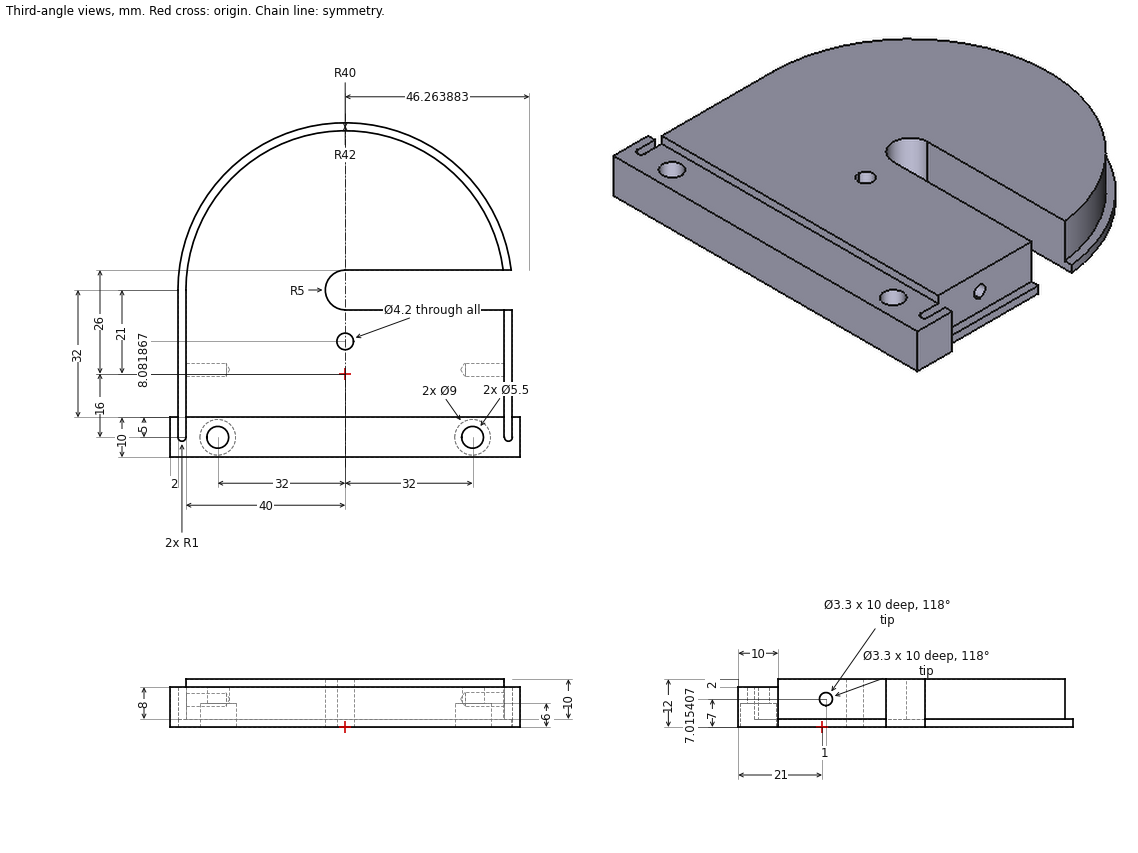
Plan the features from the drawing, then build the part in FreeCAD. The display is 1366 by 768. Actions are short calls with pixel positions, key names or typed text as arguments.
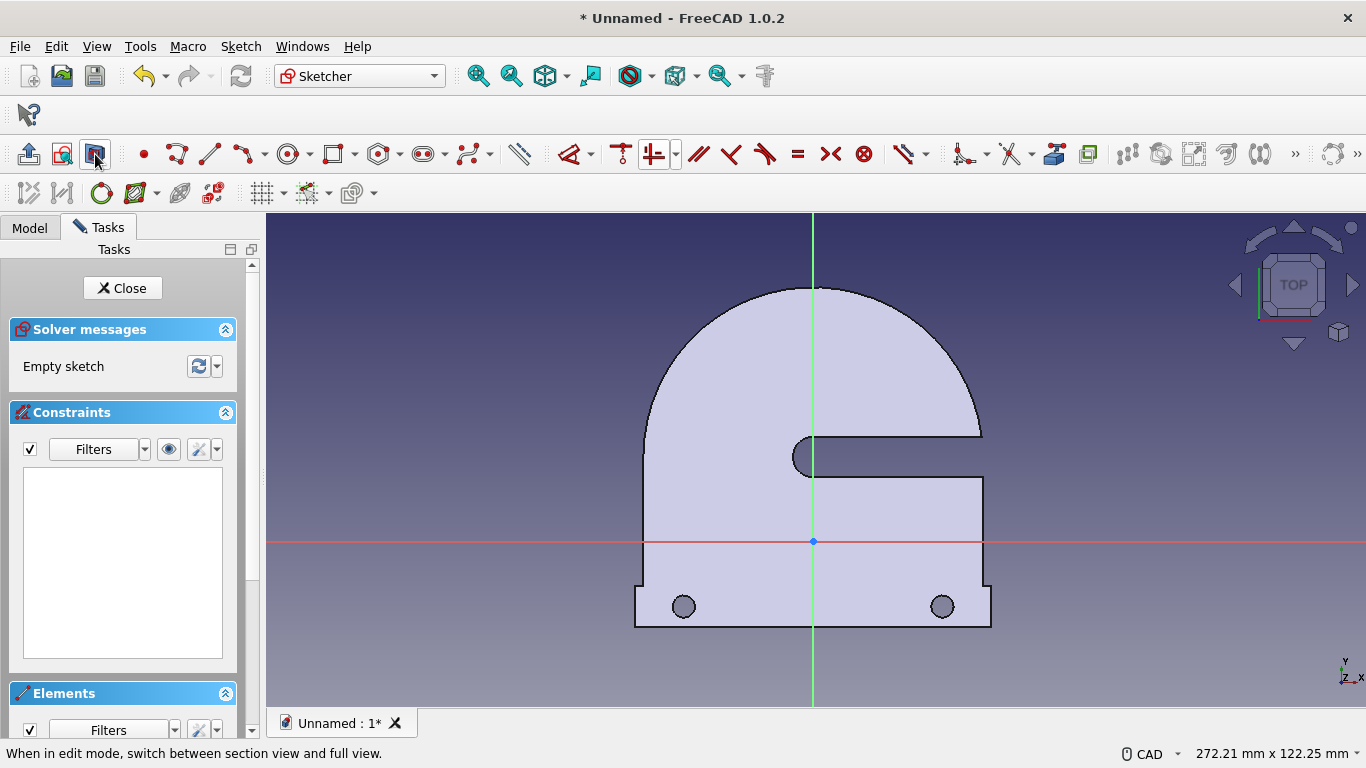
scroll(867, 679, up, 4)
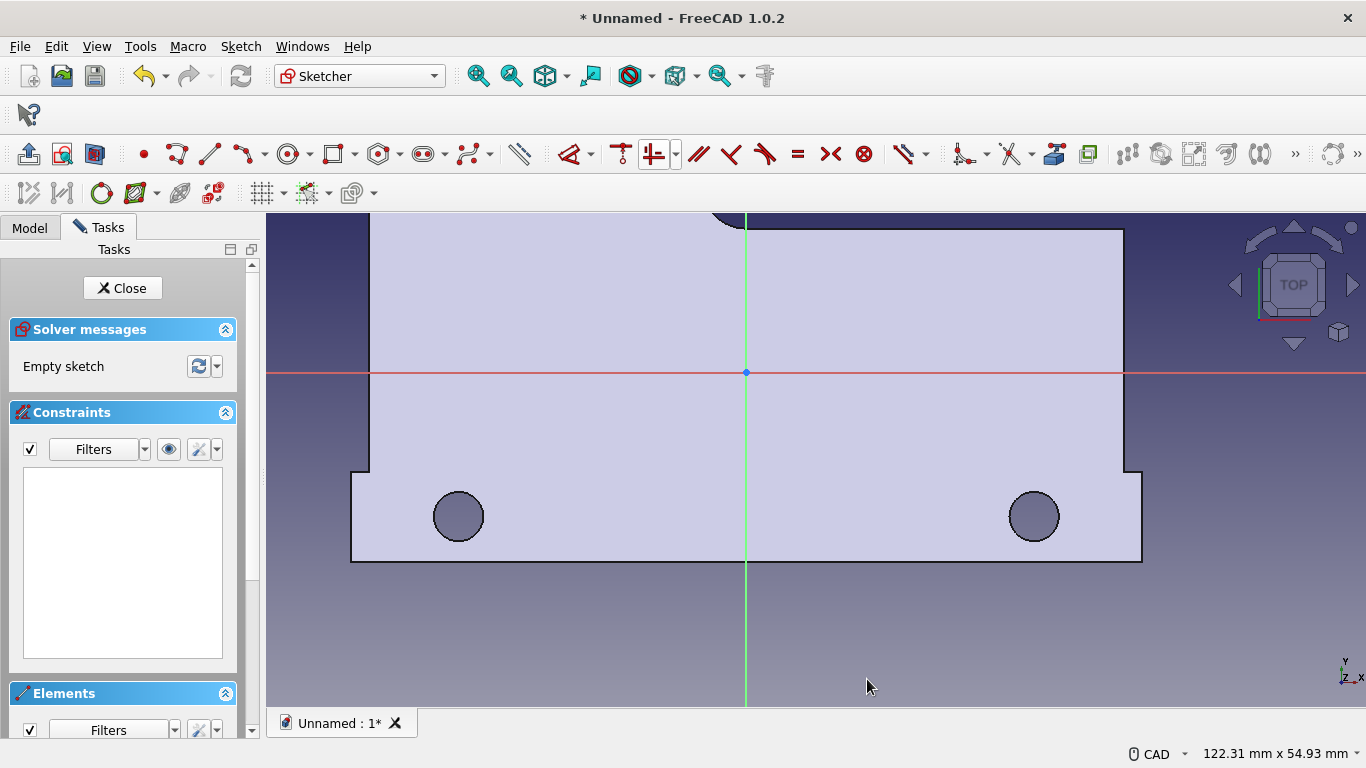
click(288, 154)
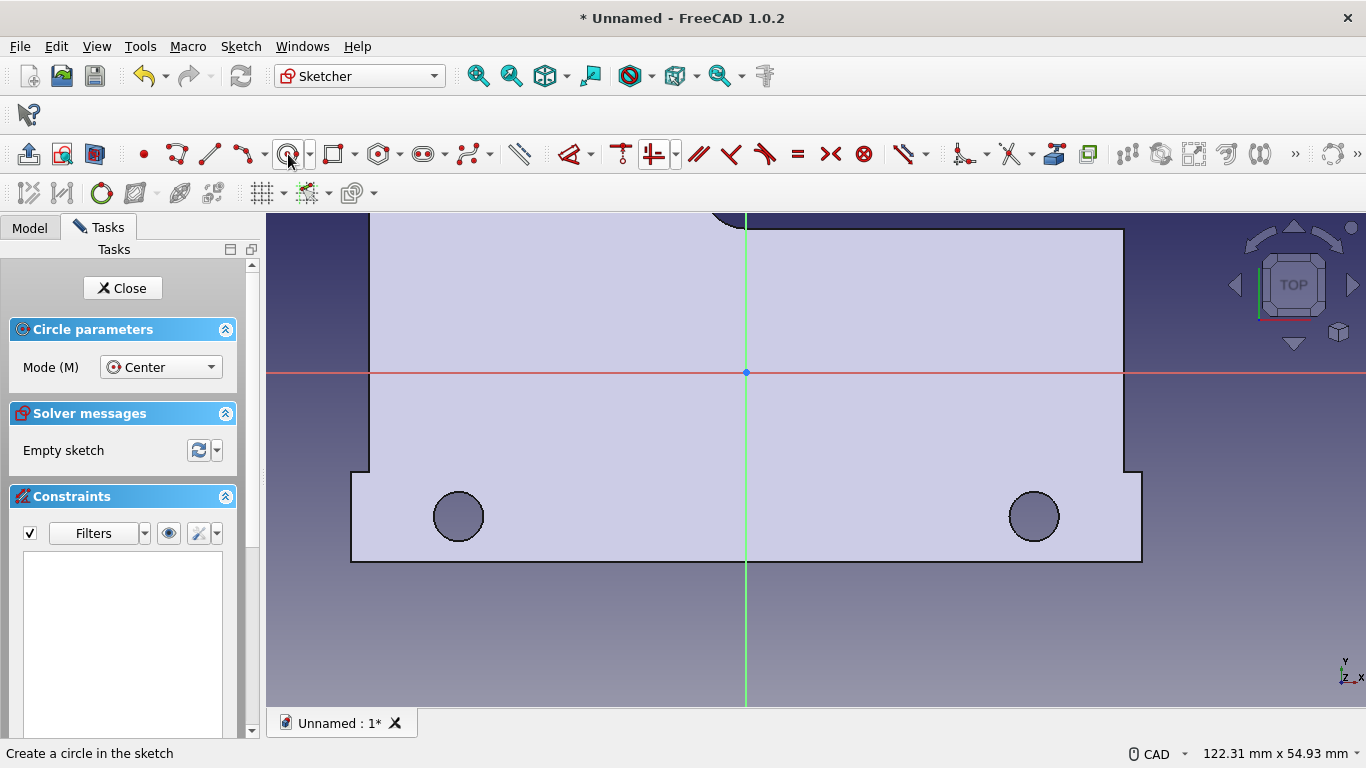
click(1034, 517)
click(1063, 488)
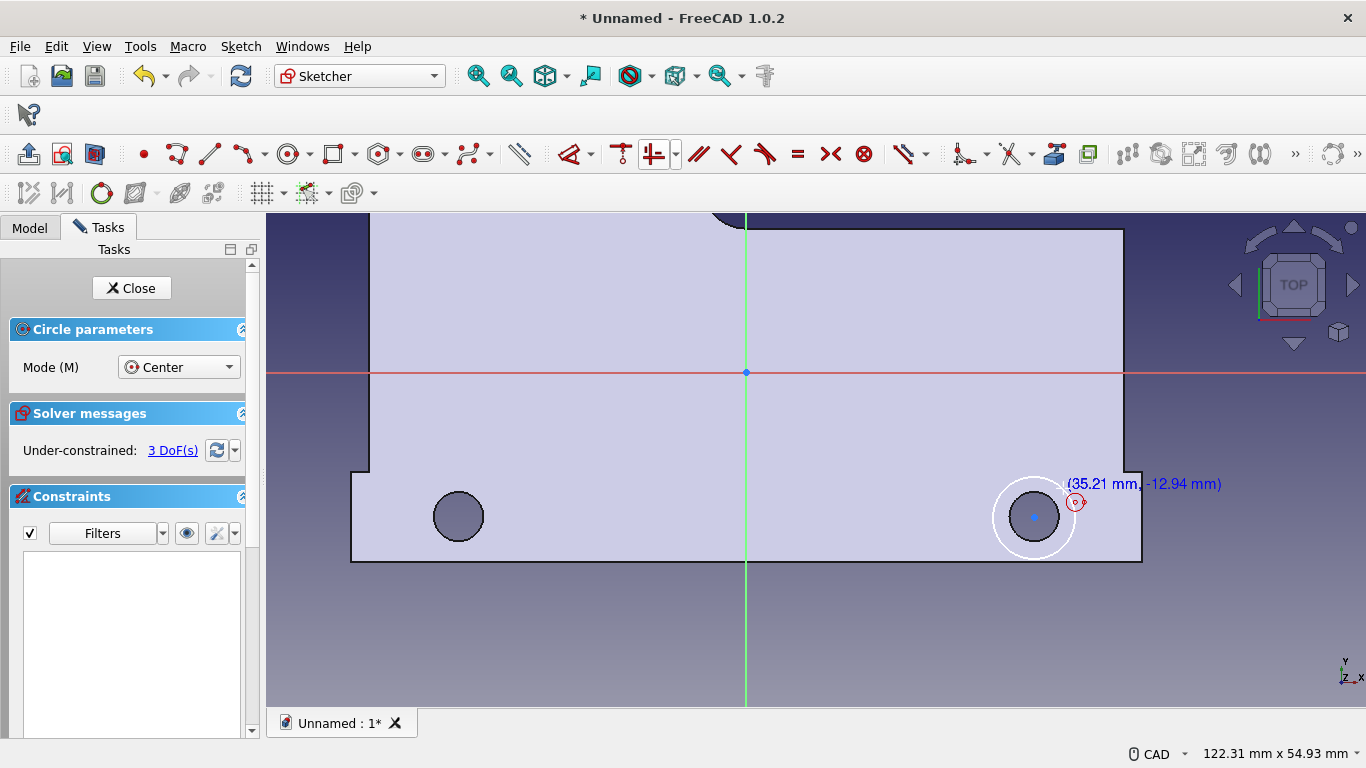
click(459, 517)
click(487, 488)
key(Escape)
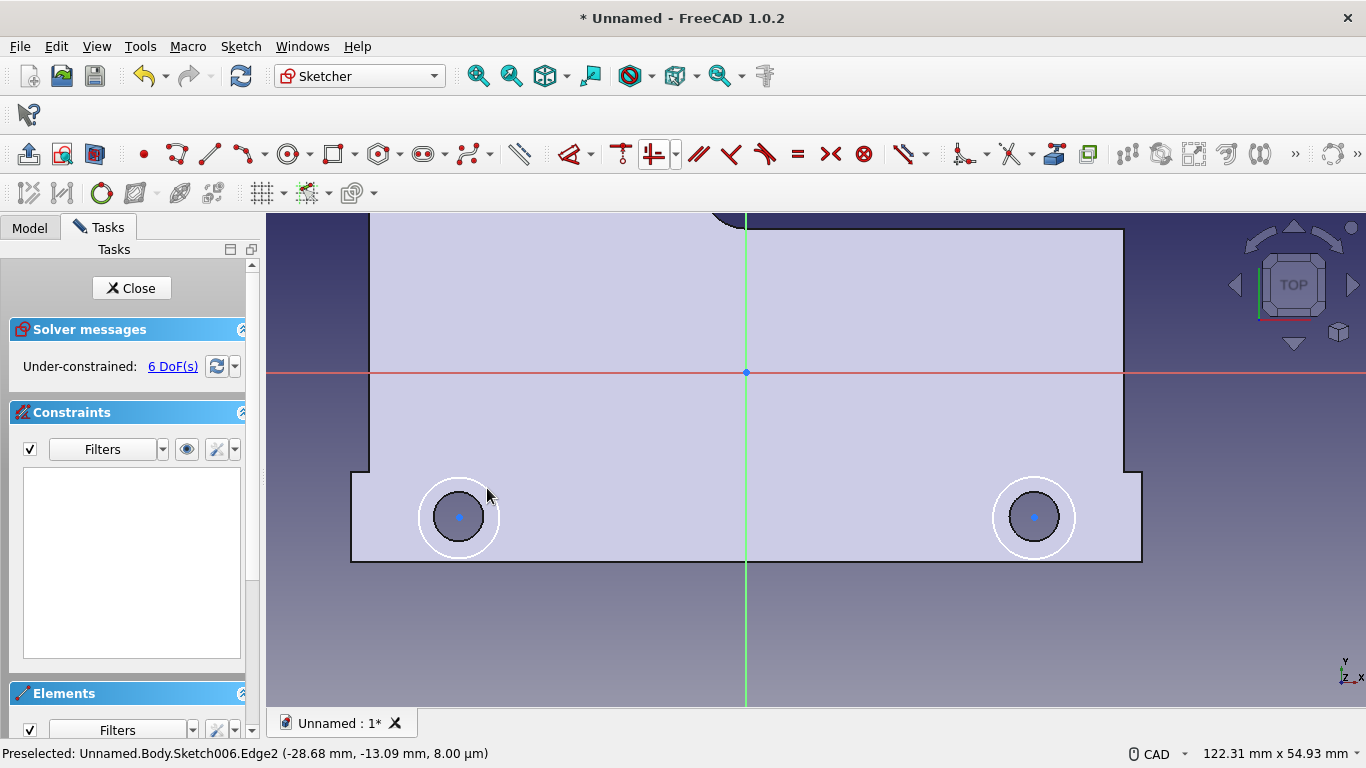
click(1063, 489)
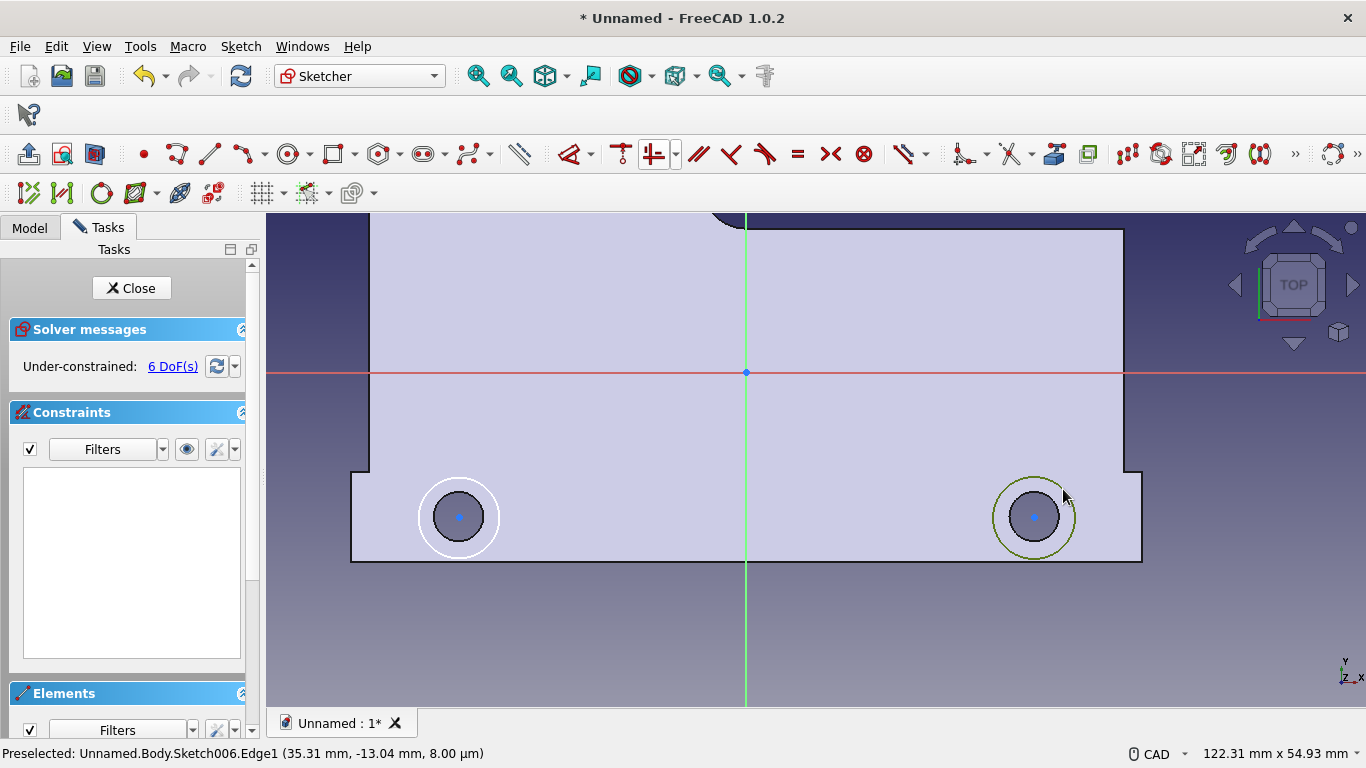
click(487, 489)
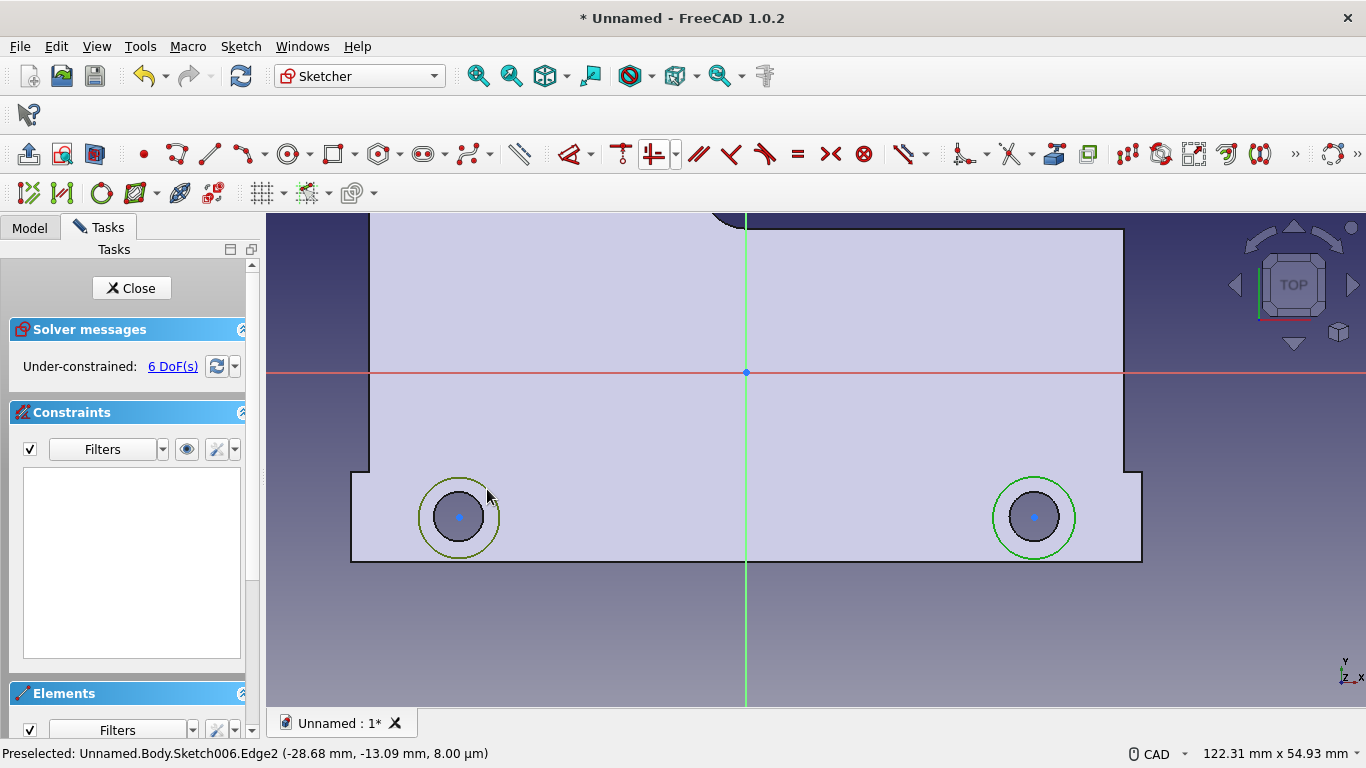
click(798, 154)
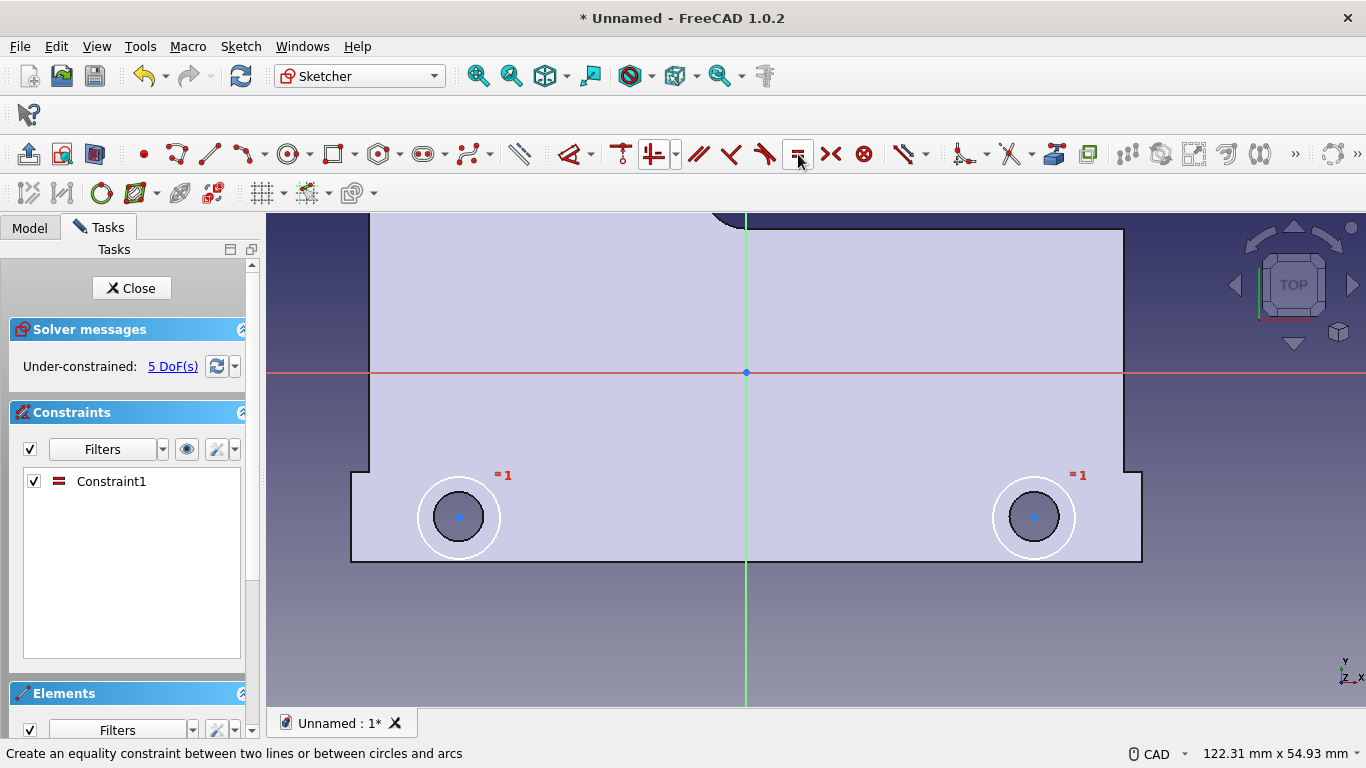
click(1034, 518)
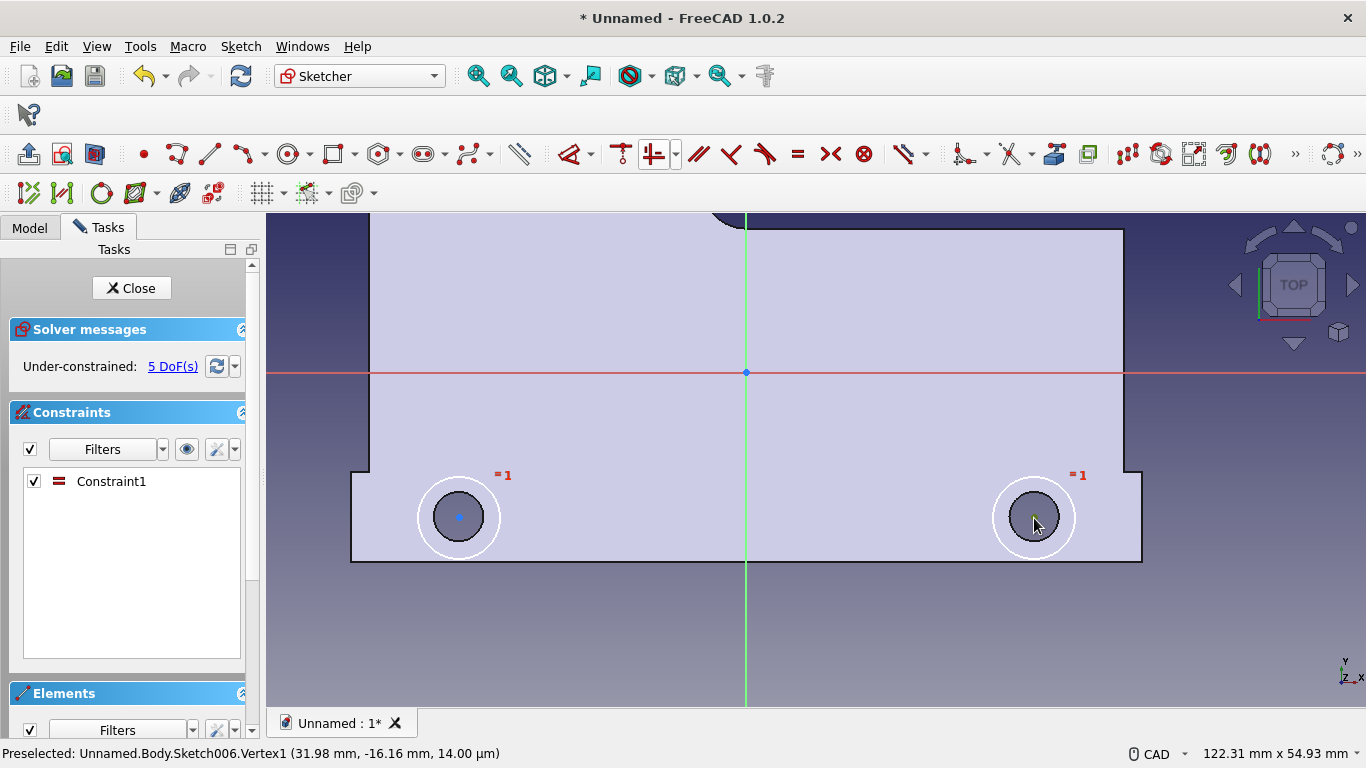
click(459, 518)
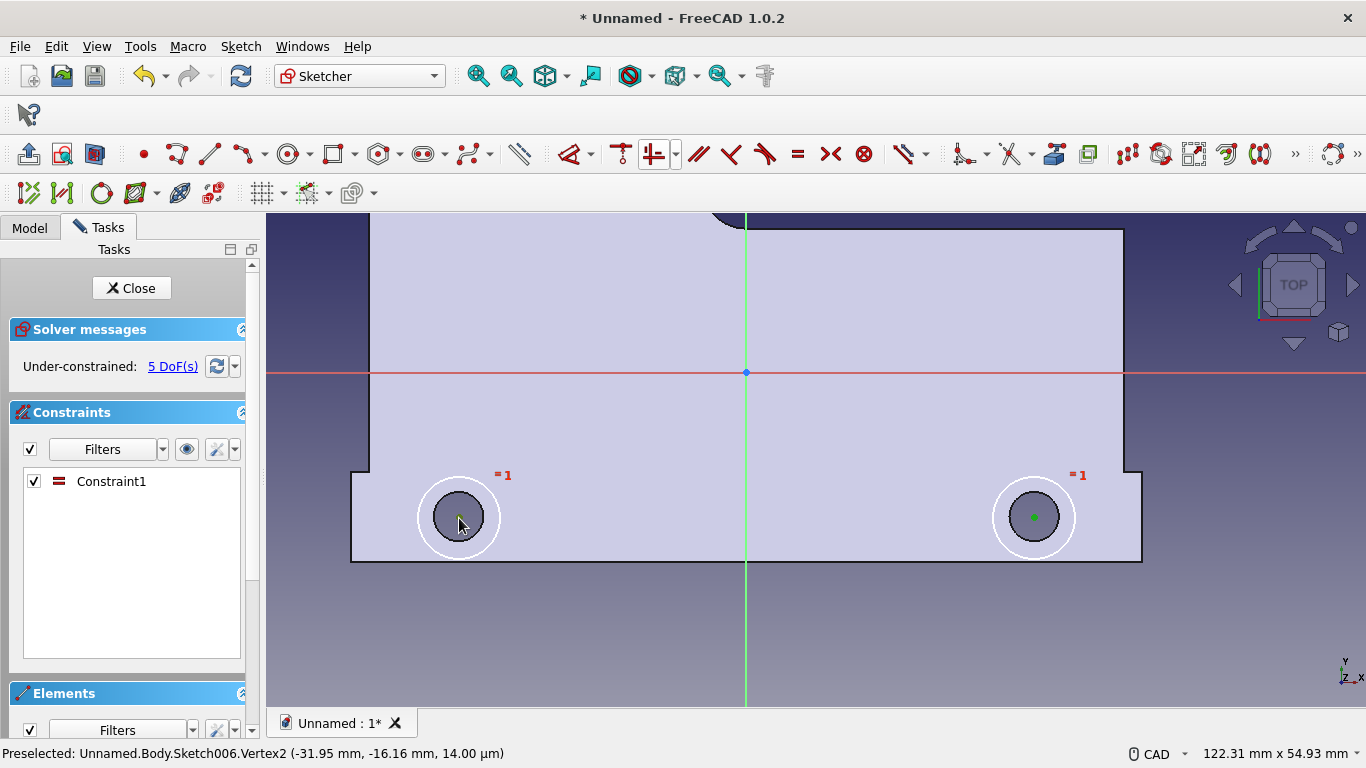
click(676, 154)